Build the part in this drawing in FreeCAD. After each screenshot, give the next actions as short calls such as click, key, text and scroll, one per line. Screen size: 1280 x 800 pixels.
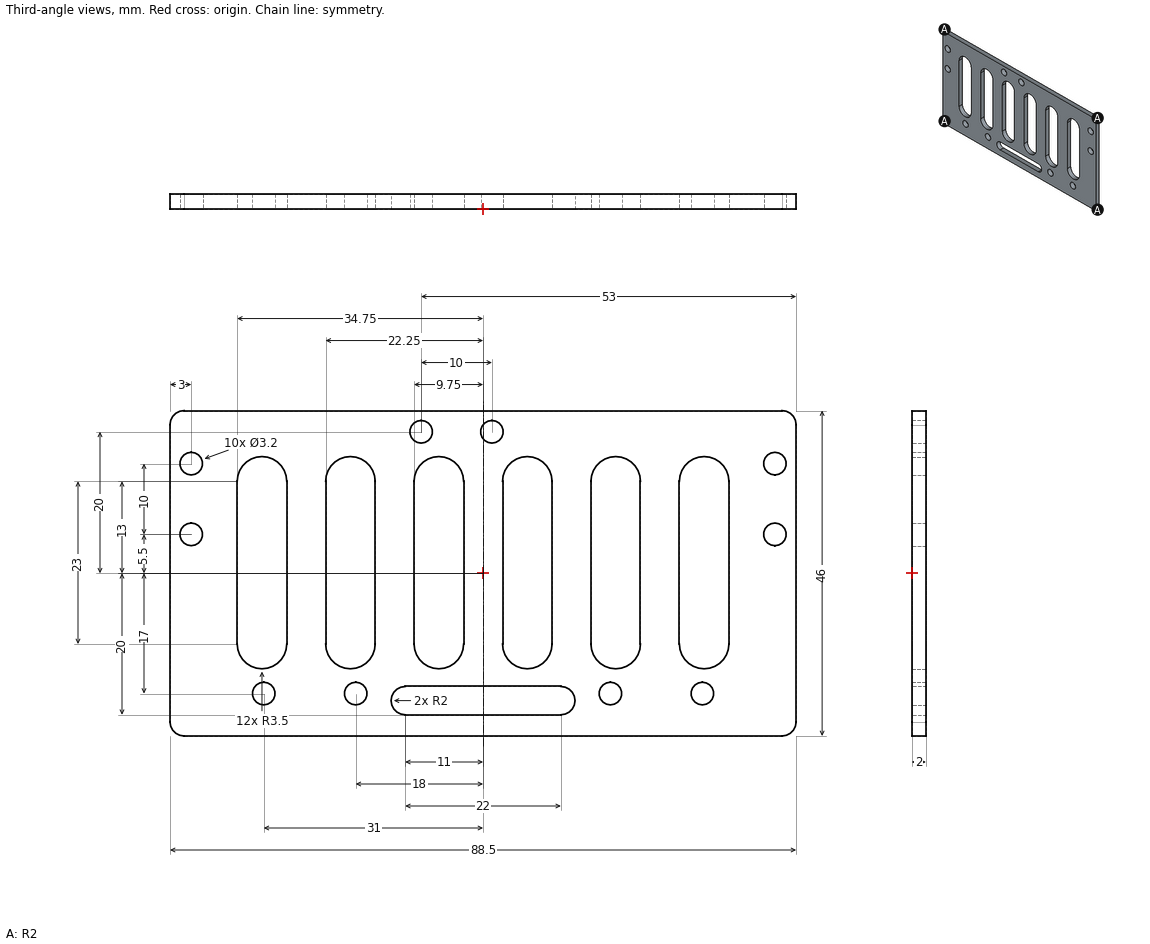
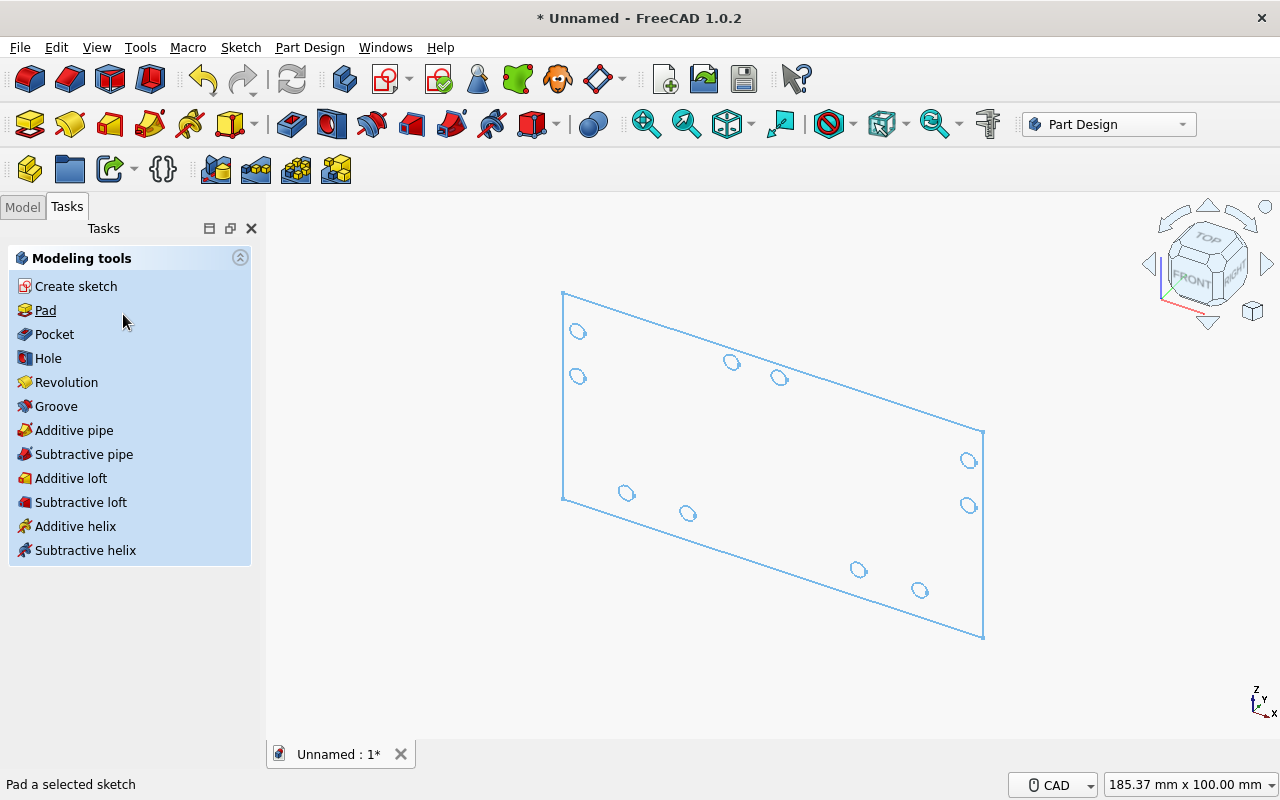
click(30, 124)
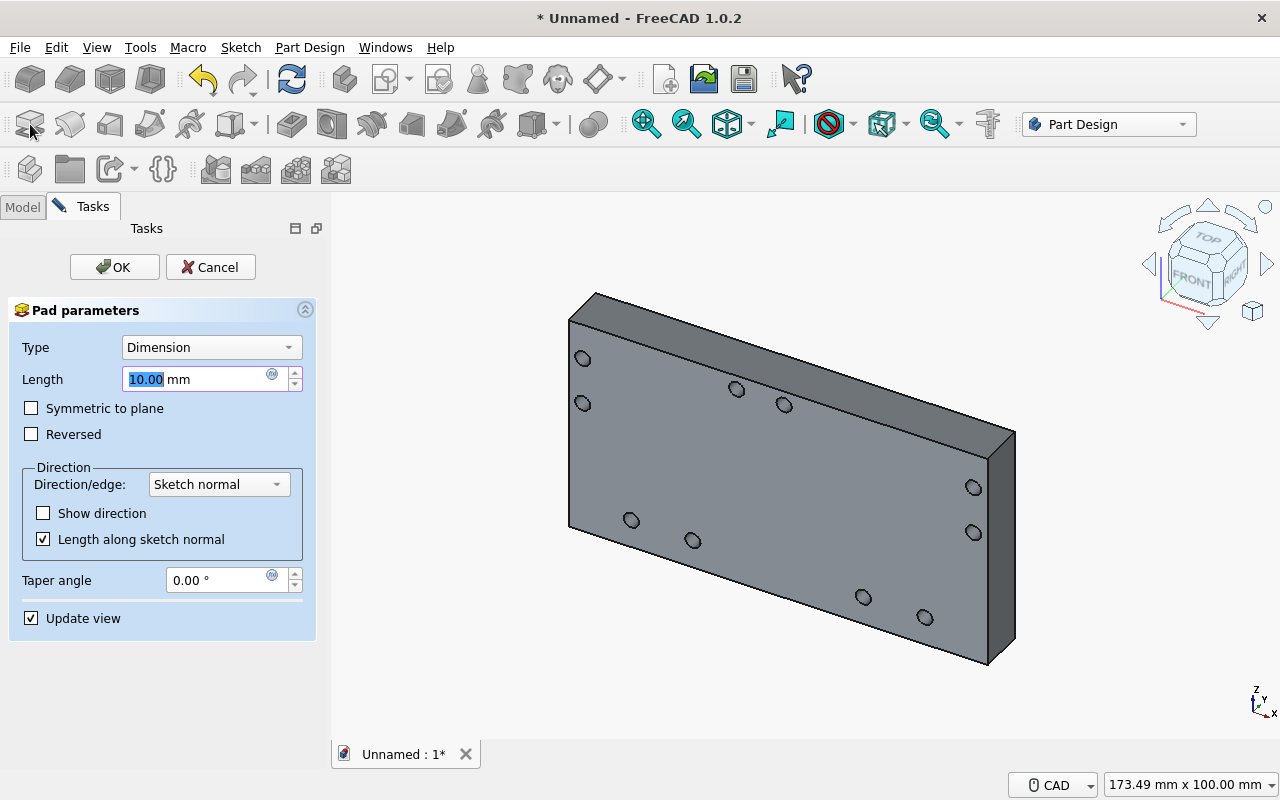
text(2)
key(Tab)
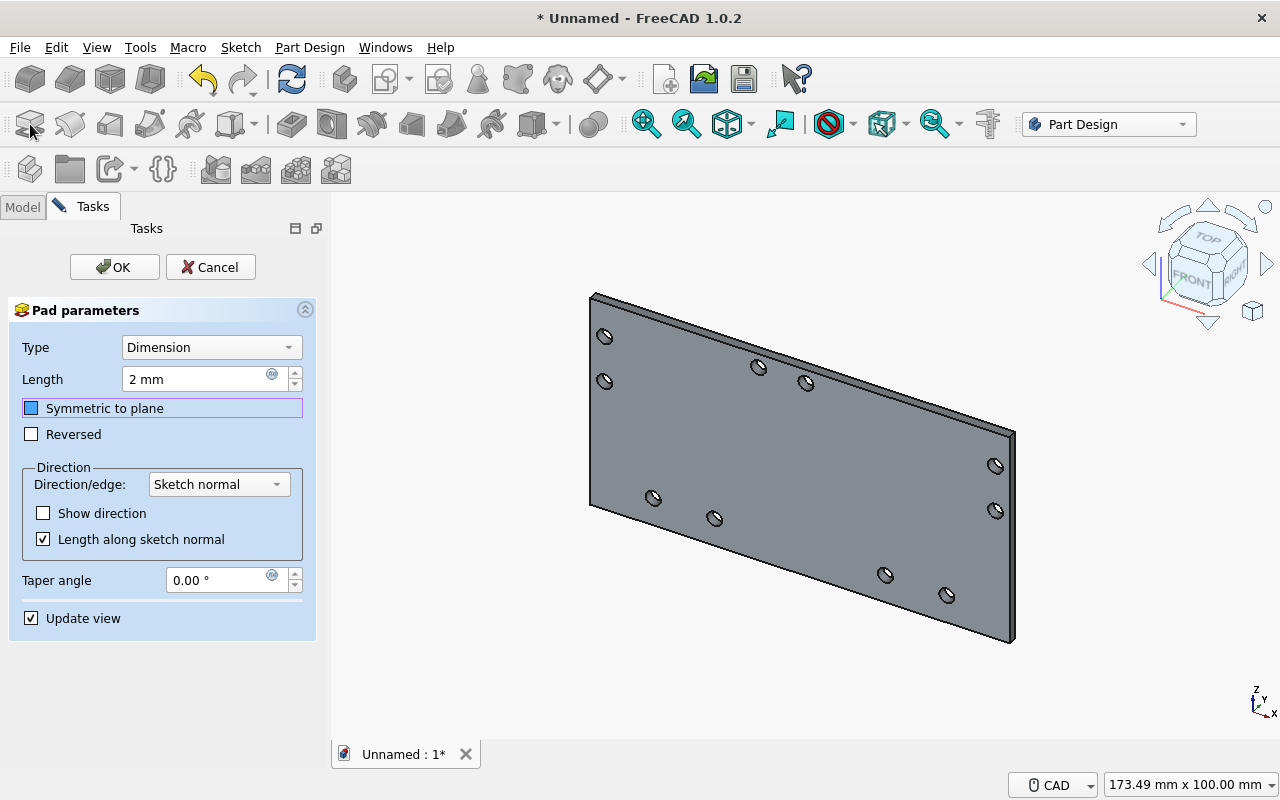
click(30, 434)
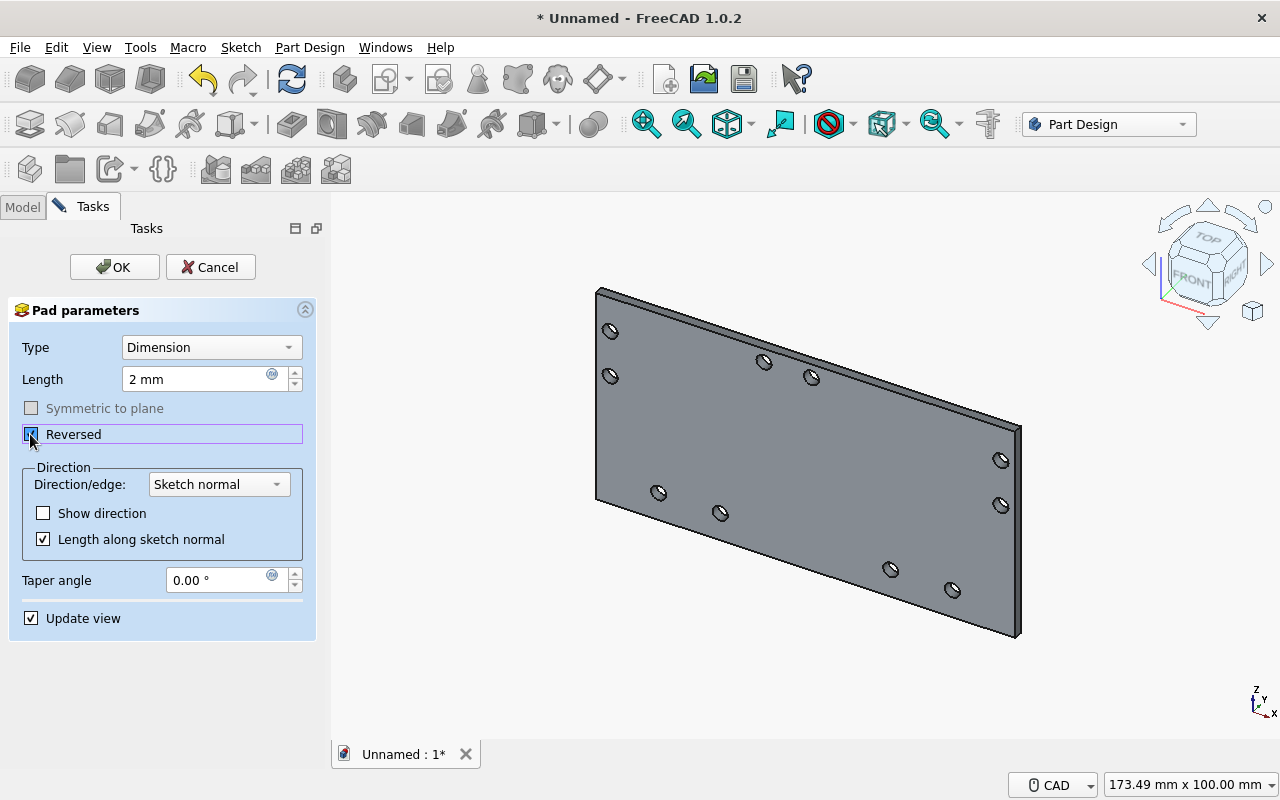
click(115, 267)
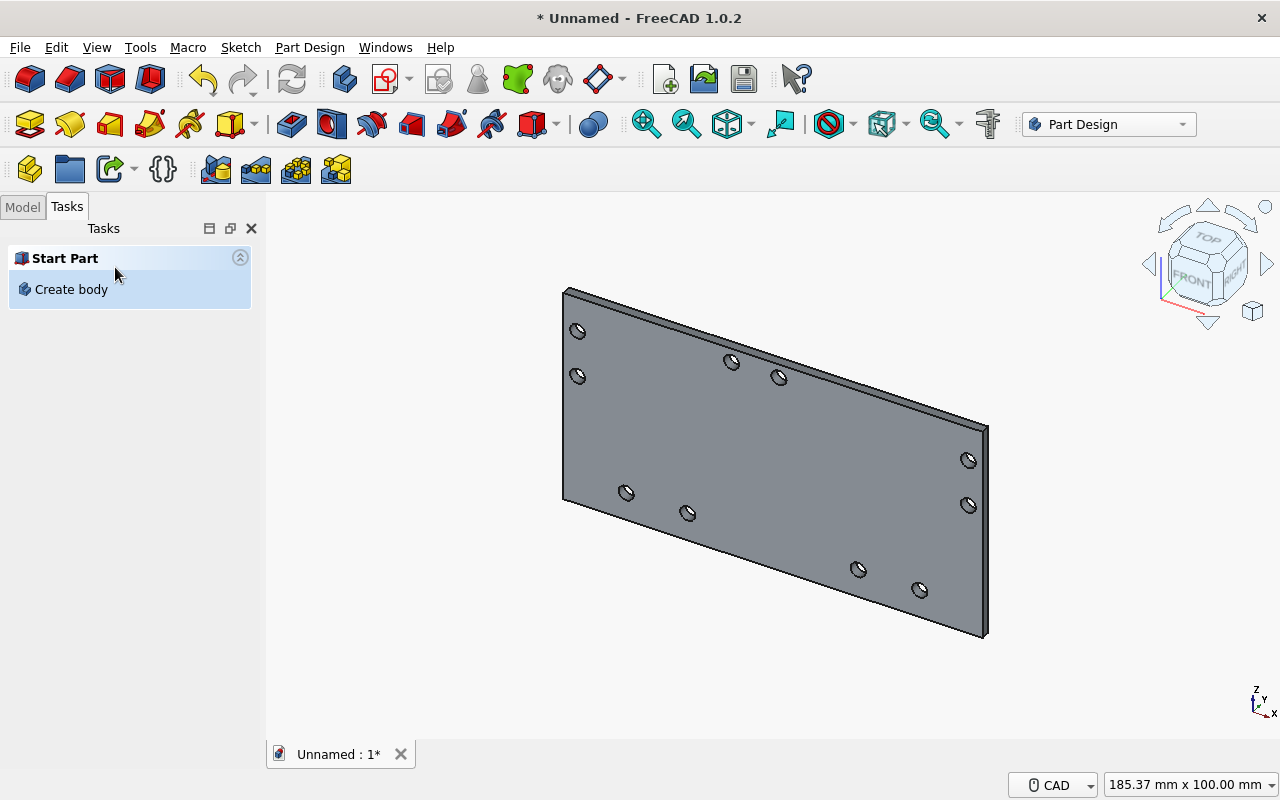
key(4)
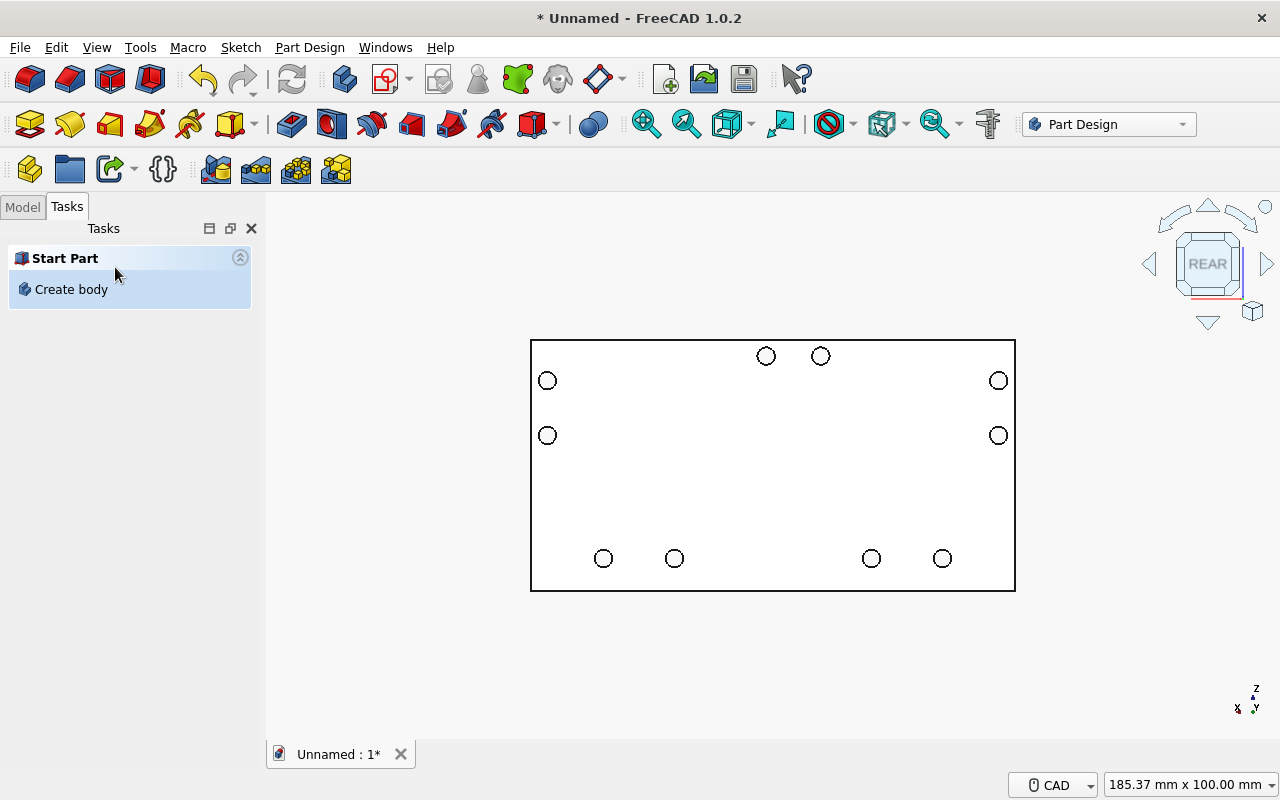
click(773, 464)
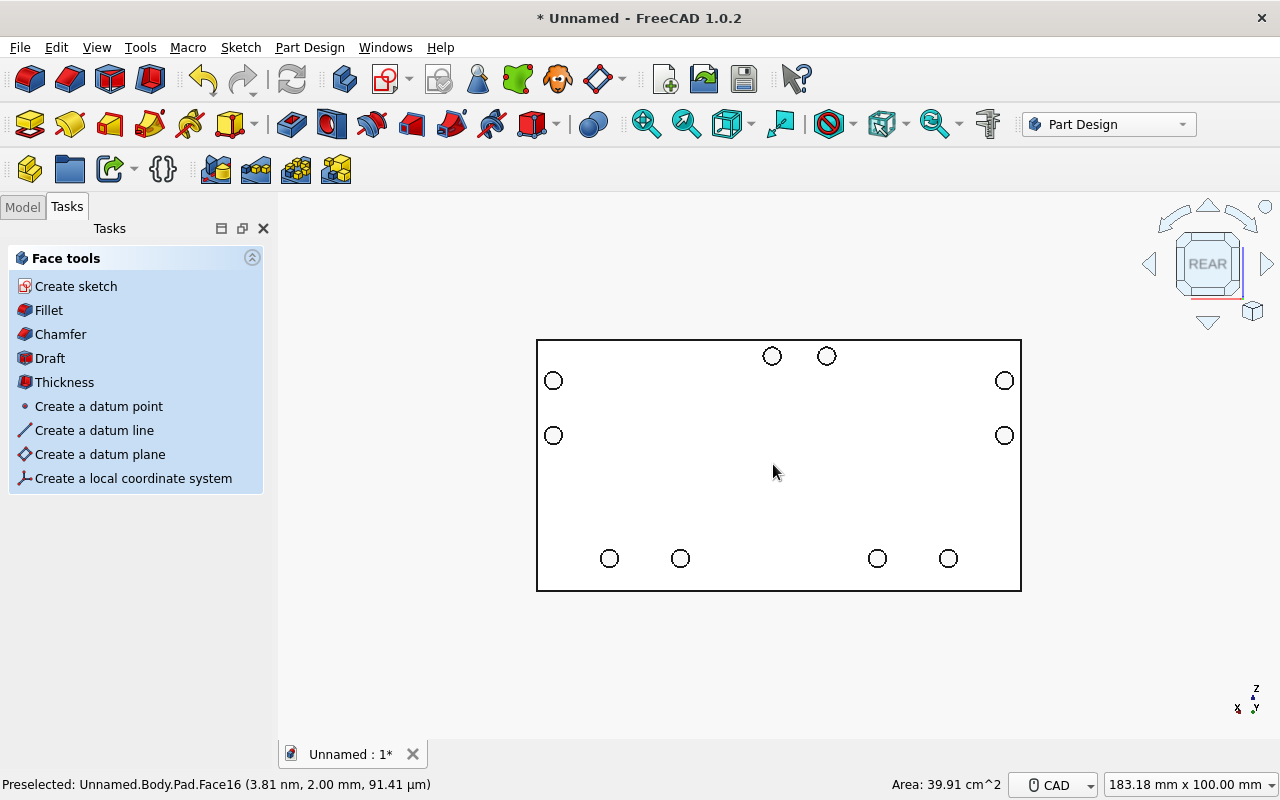
click(386, 80)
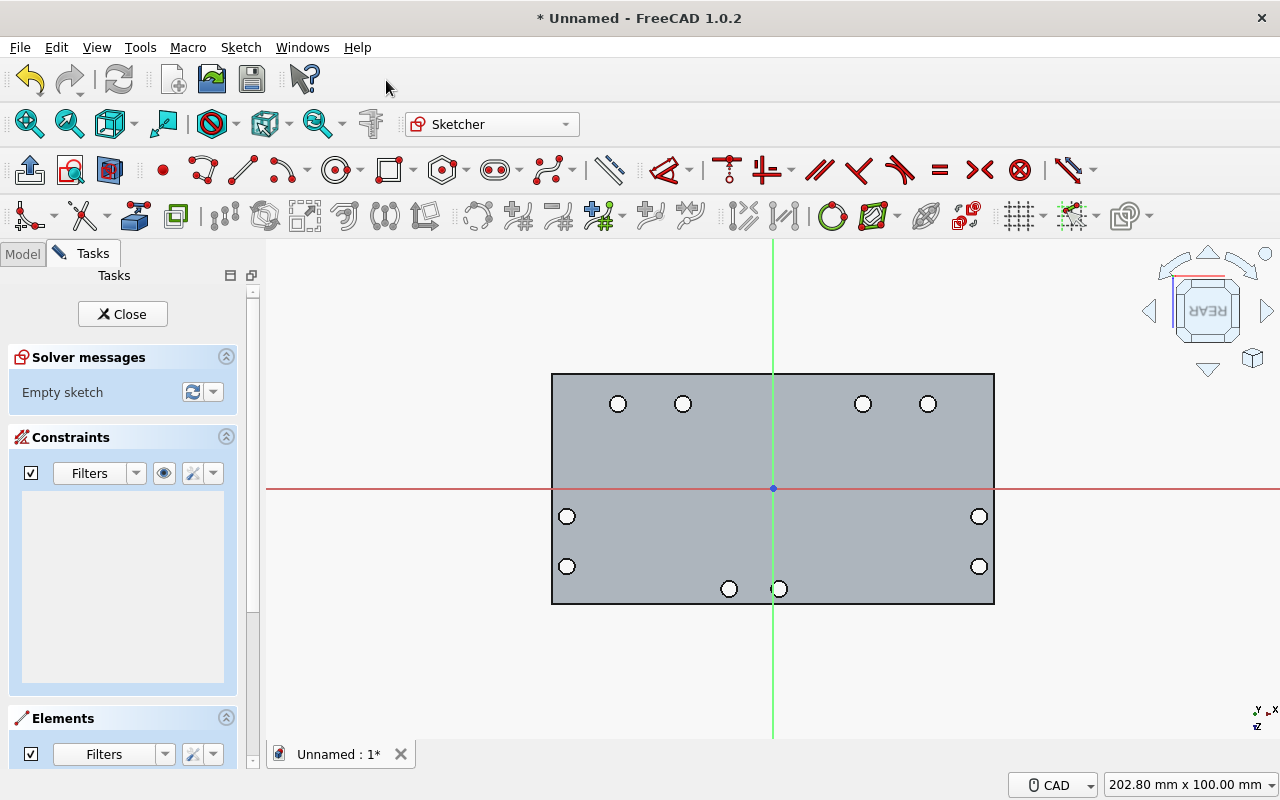
scroll(856, 470, up, 3)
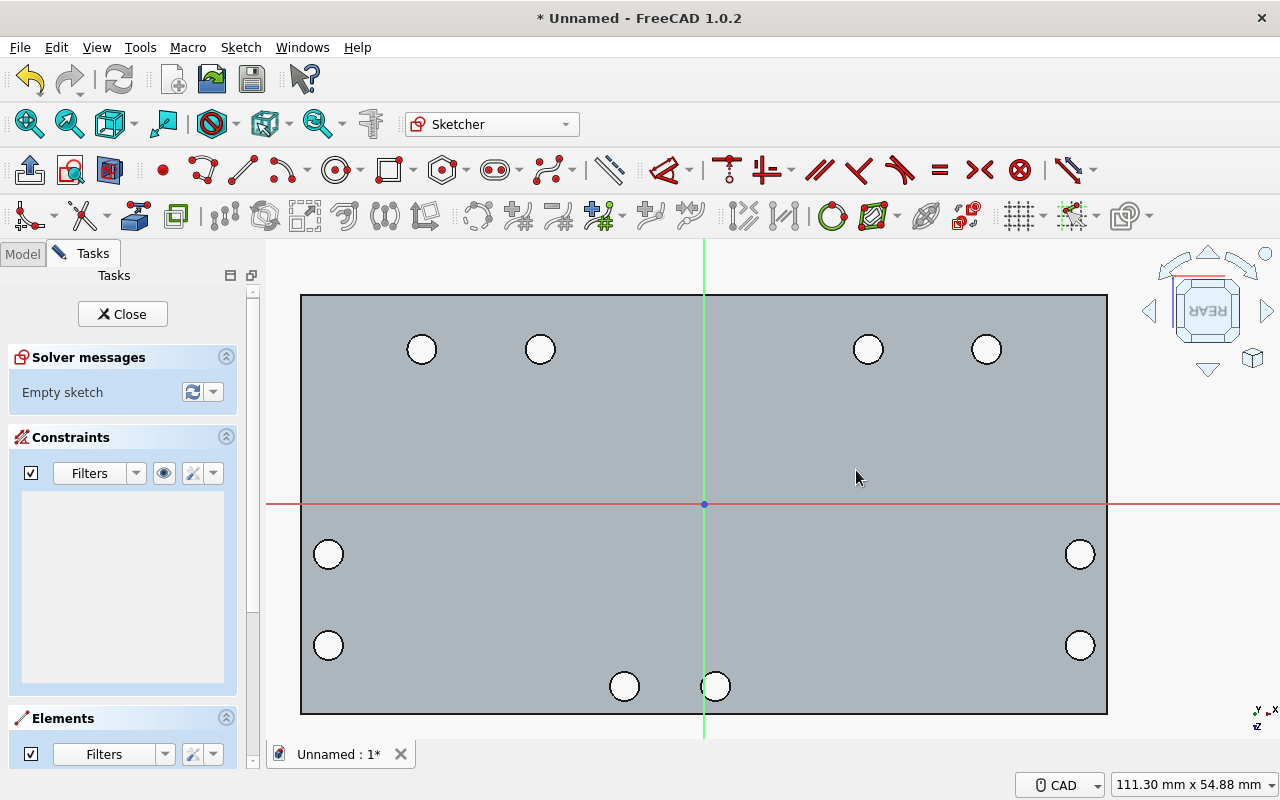
click(496, 170)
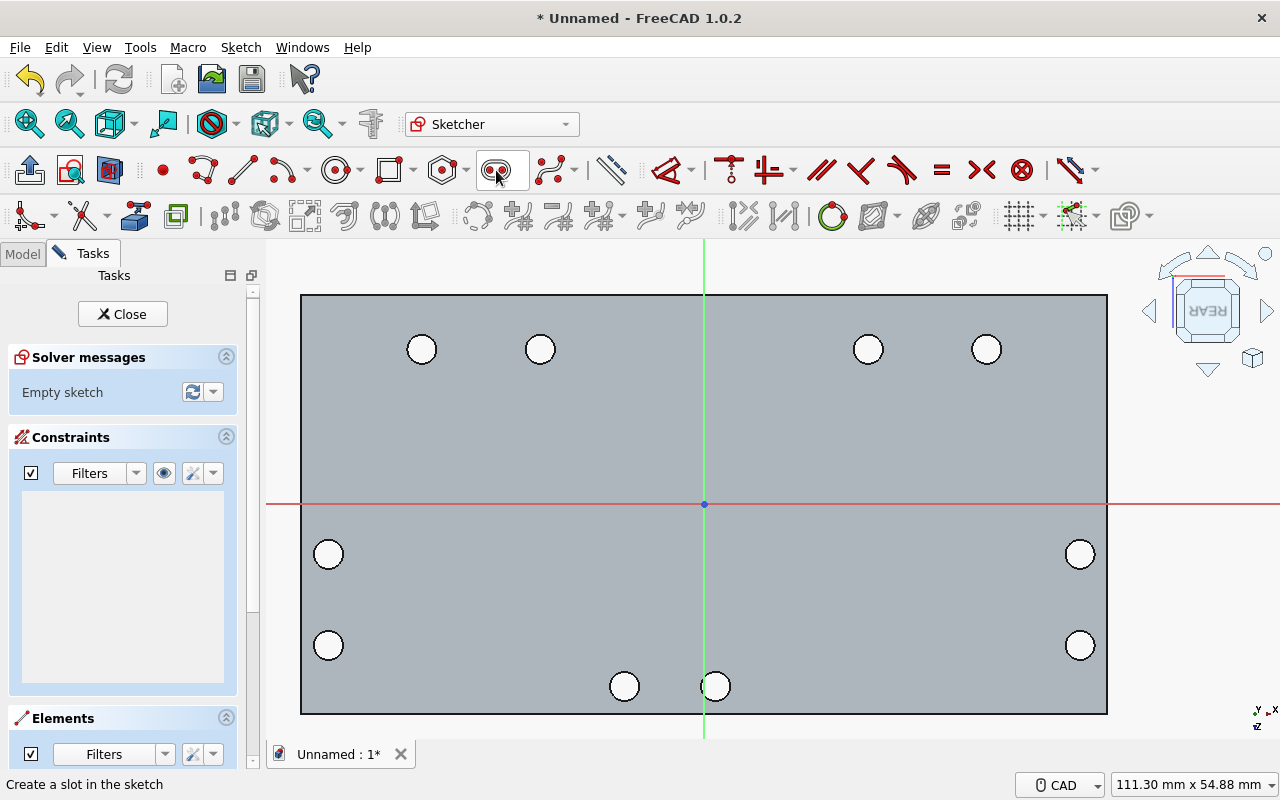
click(420, 623)